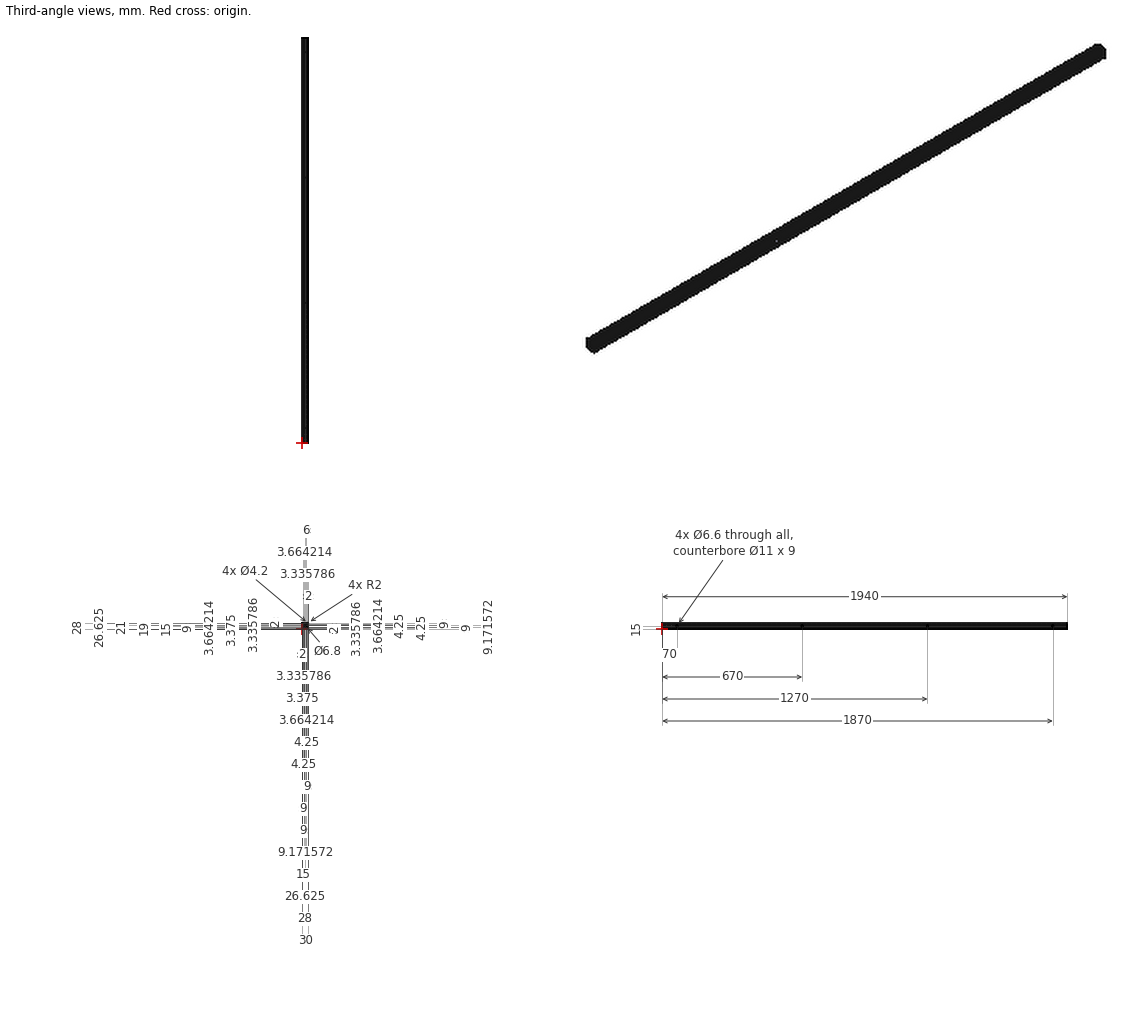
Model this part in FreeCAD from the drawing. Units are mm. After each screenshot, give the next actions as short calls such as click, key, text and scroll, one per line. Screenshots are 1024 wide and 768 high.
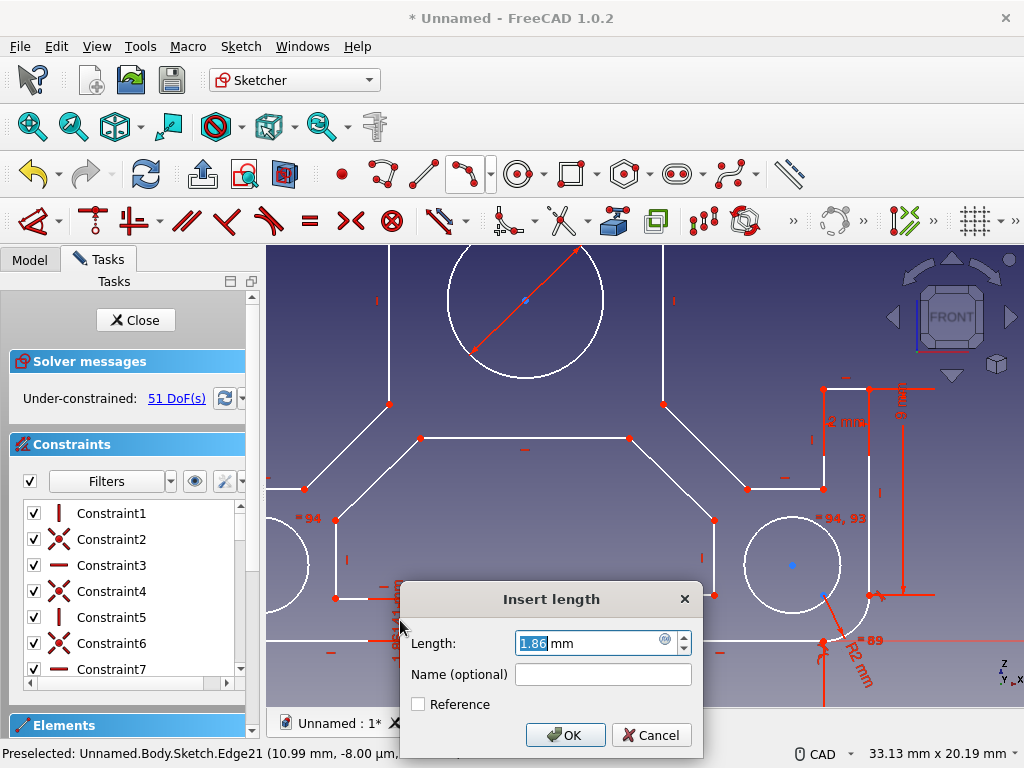
text(2)
key(Return)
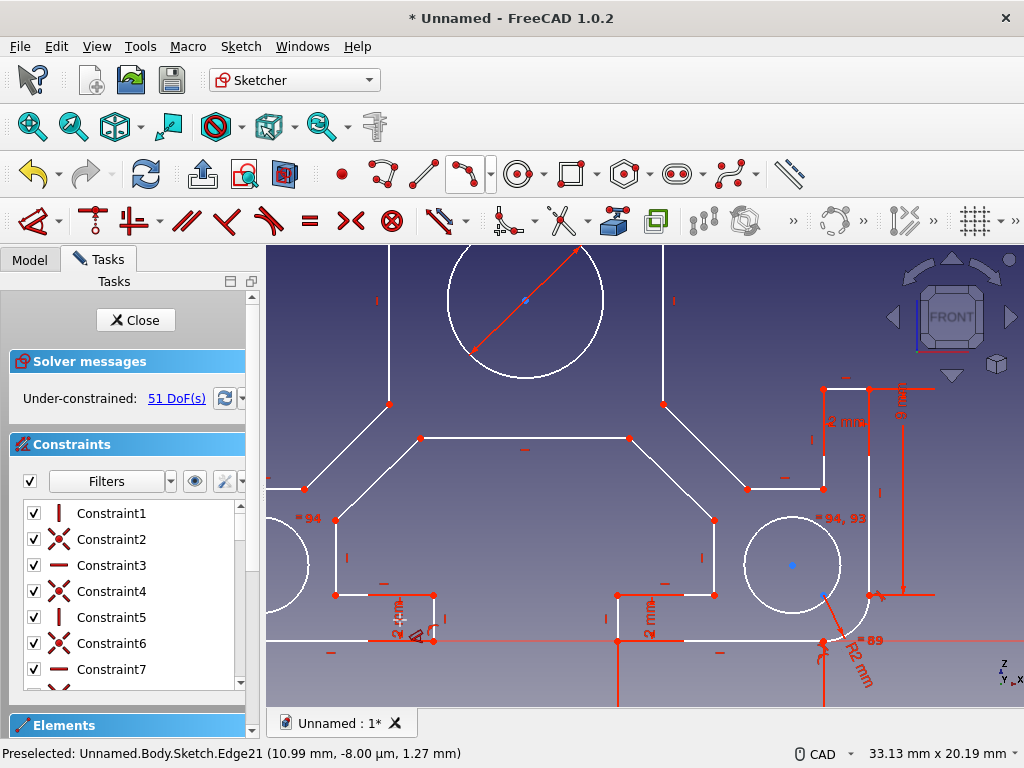
click(372, 641)
click(364, 675)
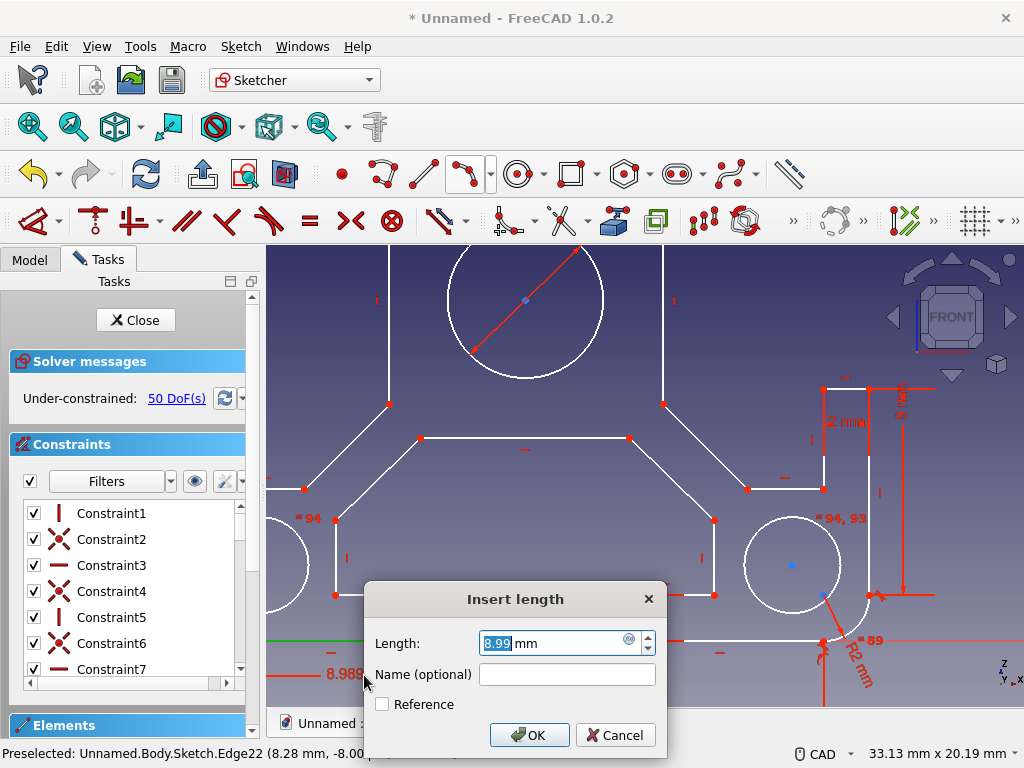
text(9)
key(Return)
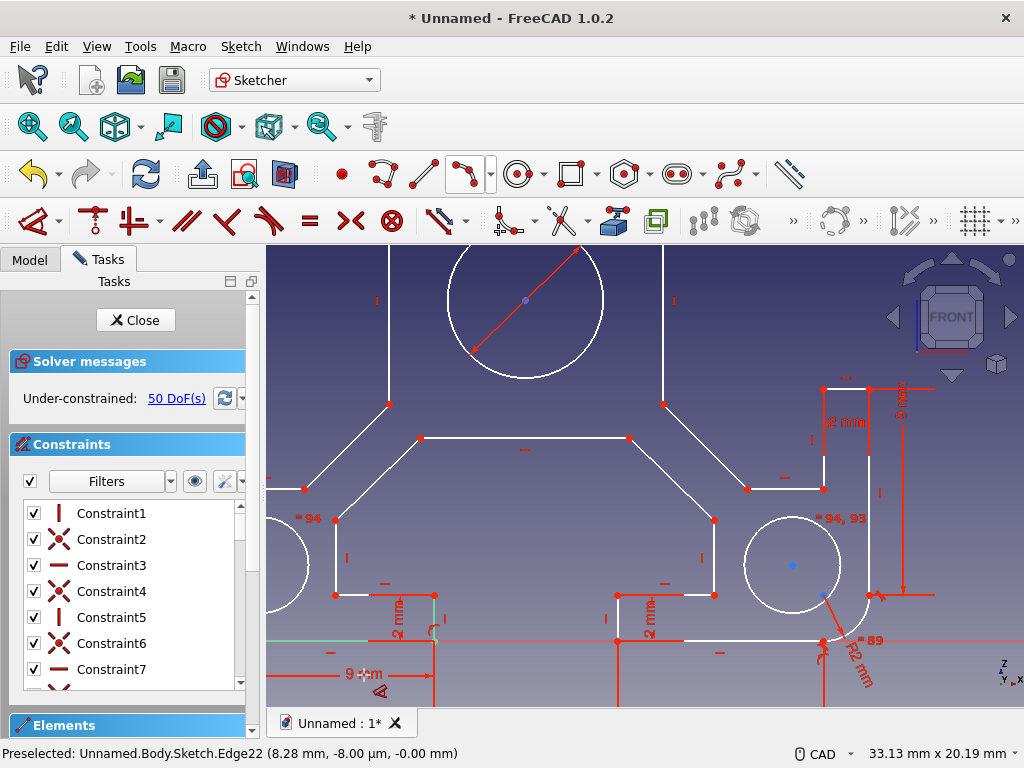
scroll(618, 621, down, 4)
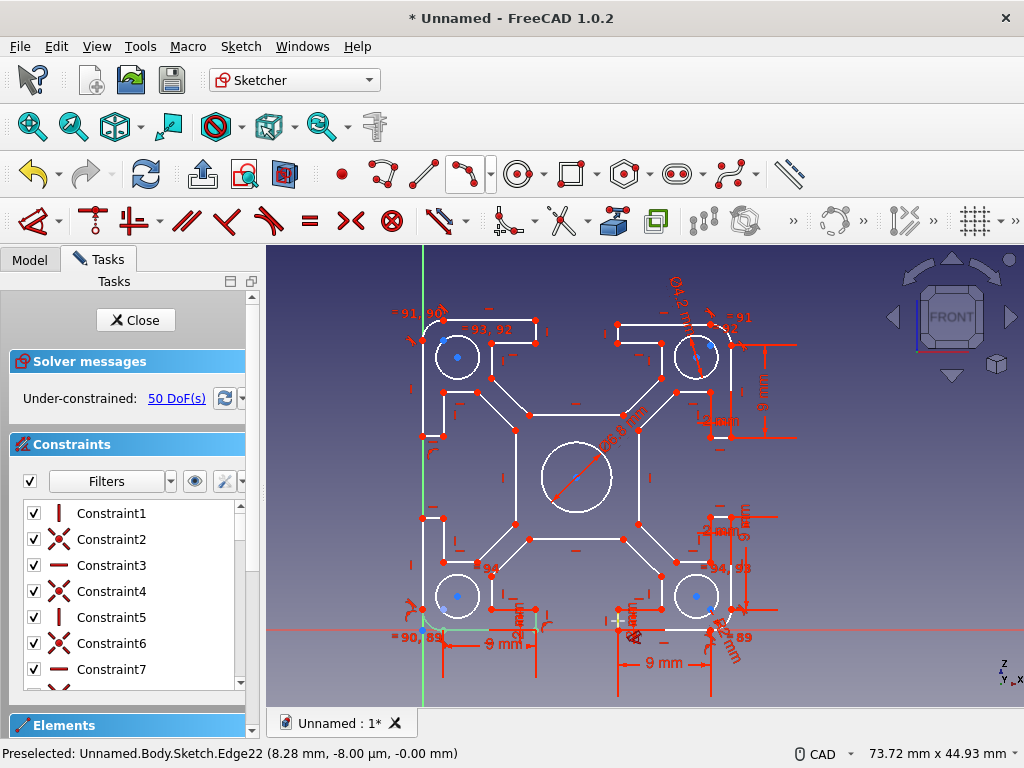
click(423, 582)
click(389, 564)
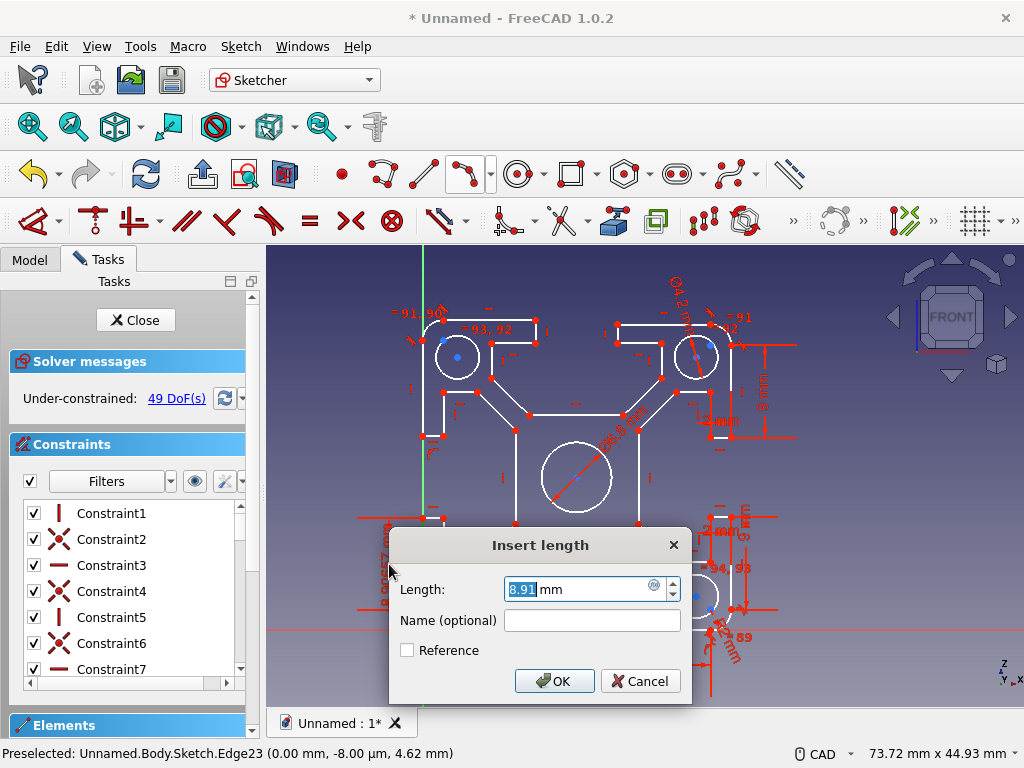
text(9)
key(Return)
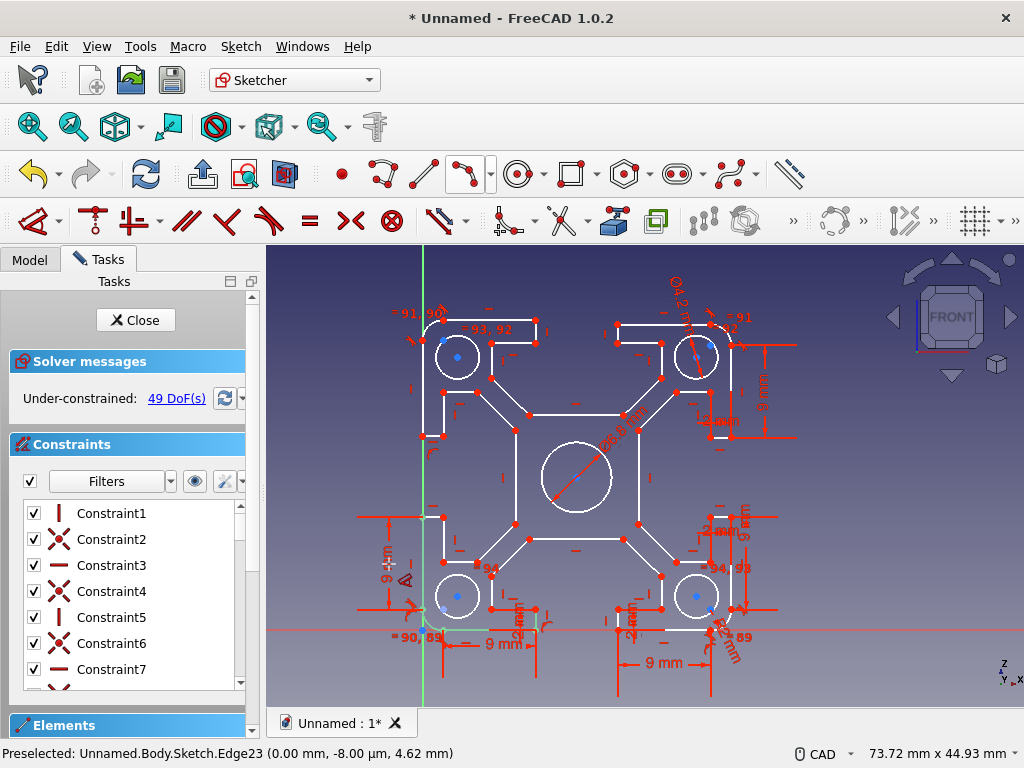
scroll(433, 517, up, 4)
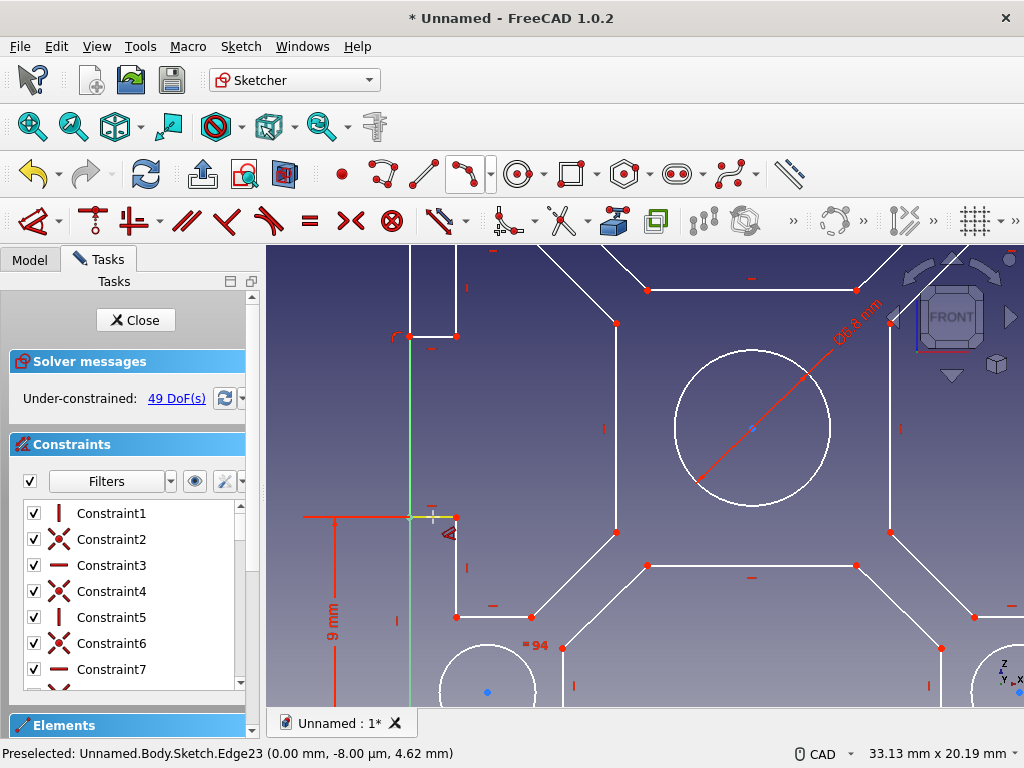
click(433, 517)
click(433, 551)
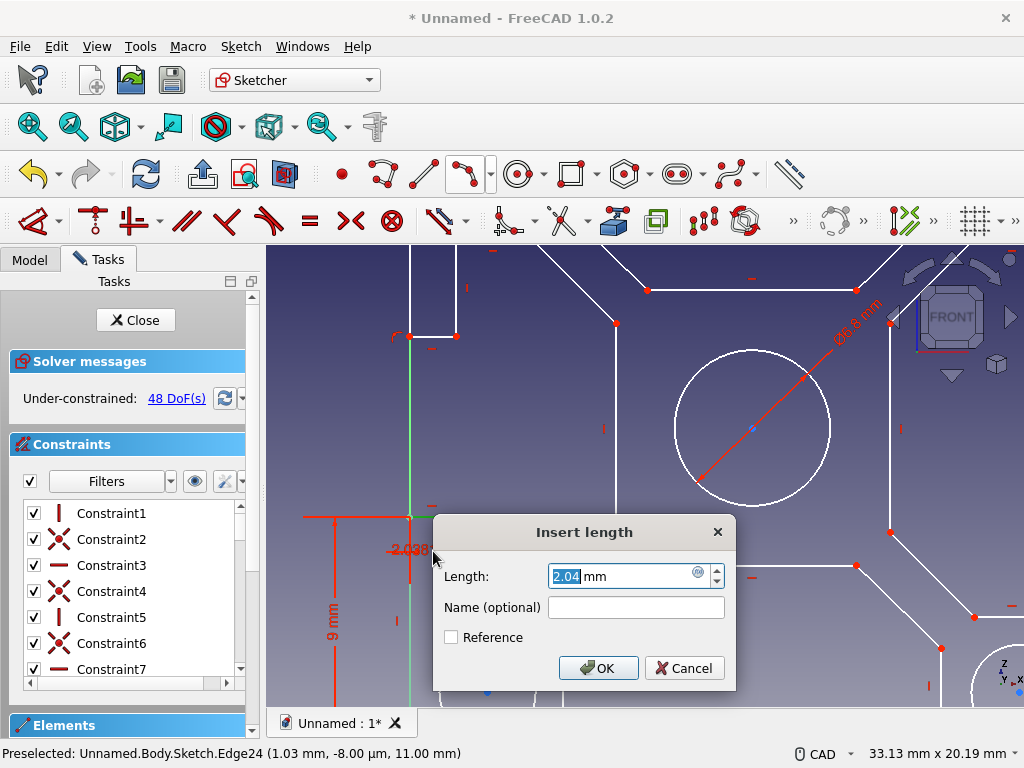
text(2)
key(Return)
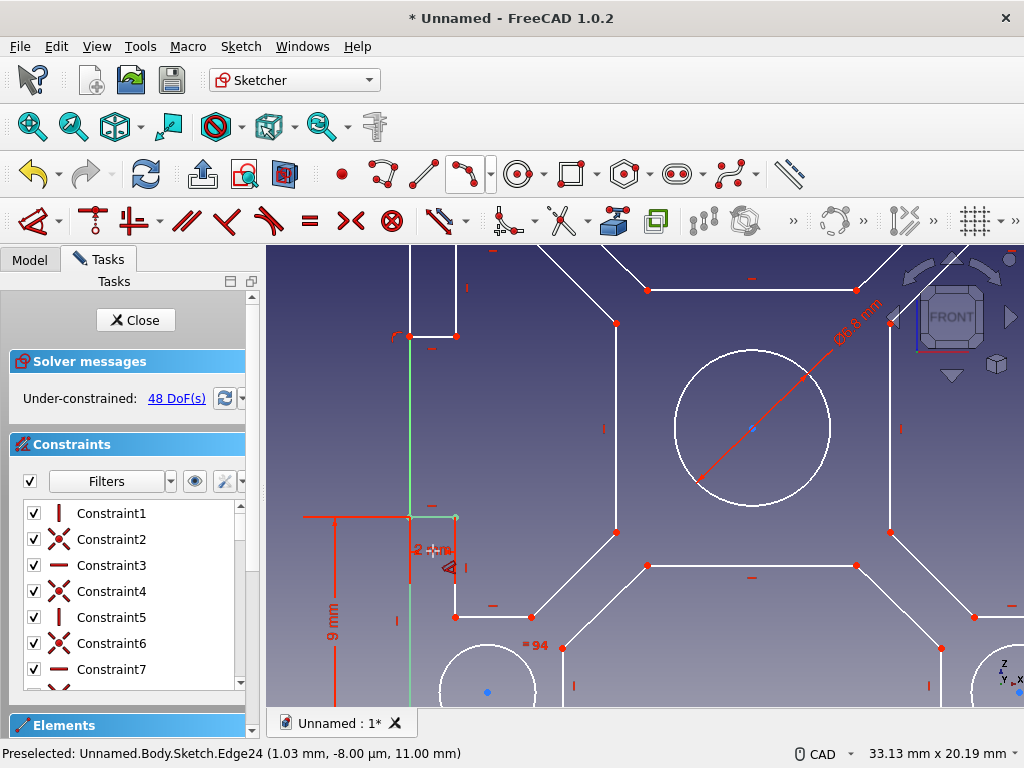
click(442, 337)
click(433, 303)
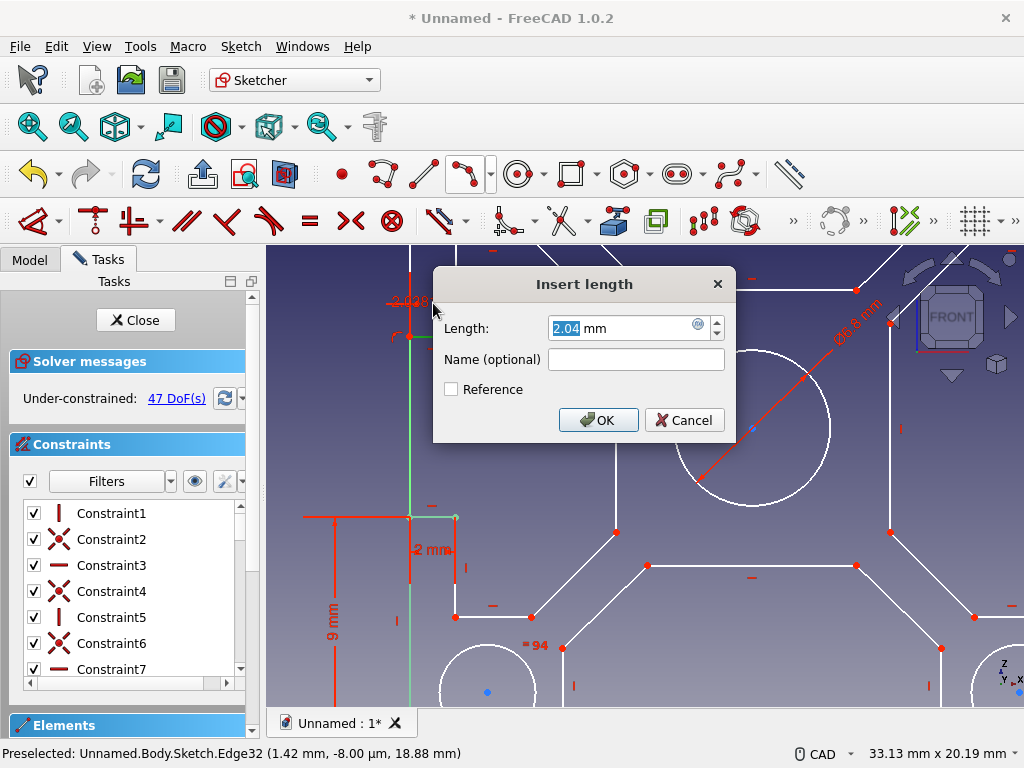
text(2)
key(Return)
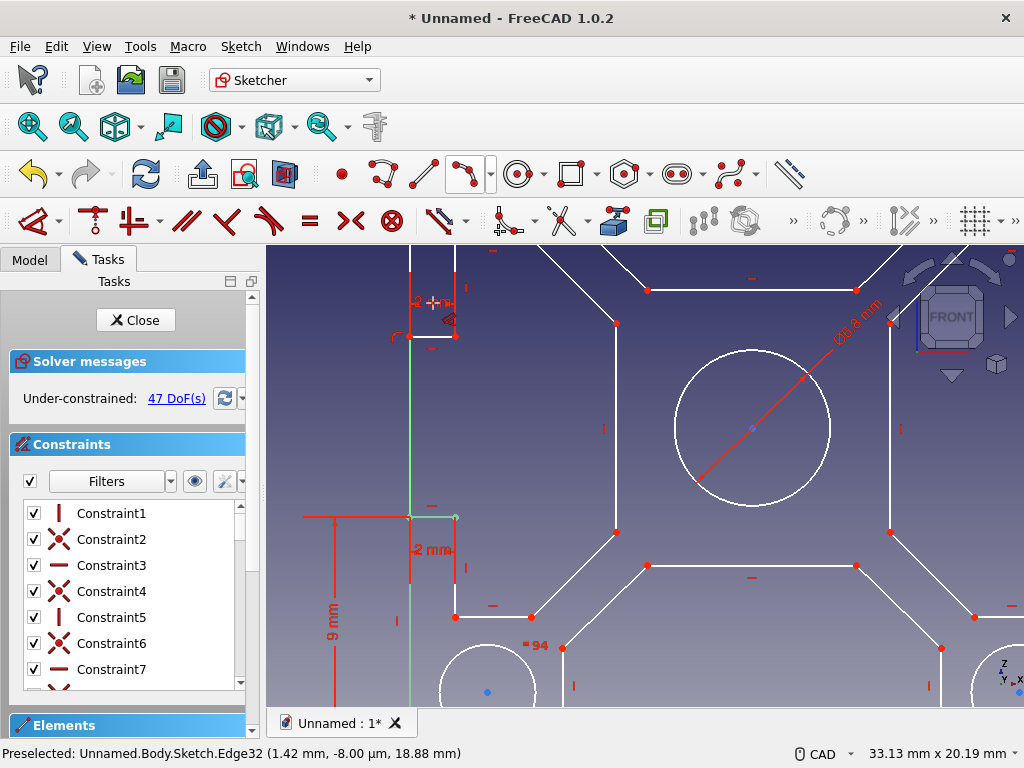
click(410, 273)
click(376, 283)